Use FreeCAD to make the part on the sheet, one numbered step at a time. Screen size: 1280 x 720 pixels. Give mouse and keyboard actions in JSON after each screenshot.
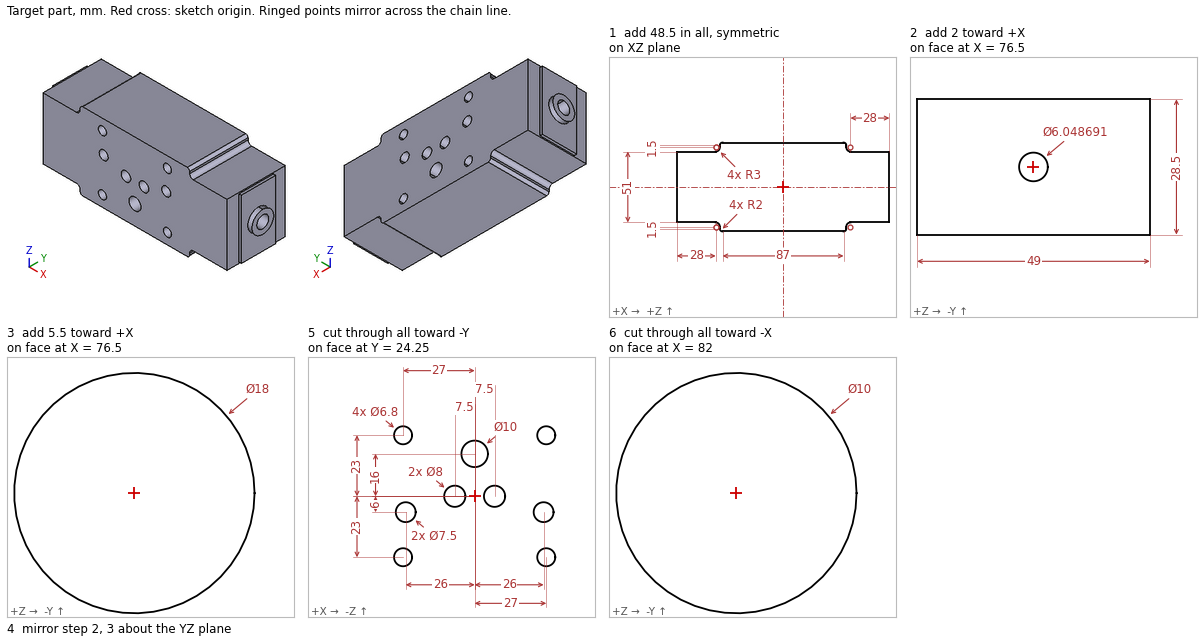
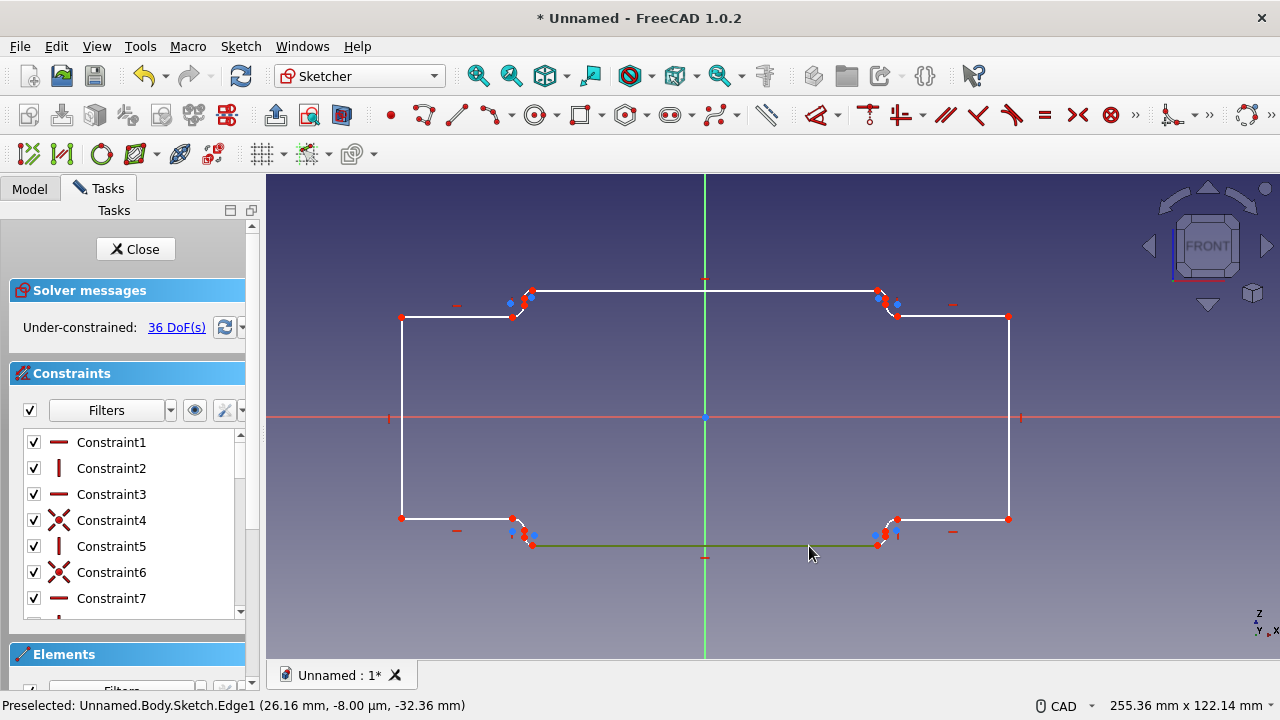
{"action": "scroll", "coordinate": [527, 543], "scroll_direction": "up", "scroll_amount": 4}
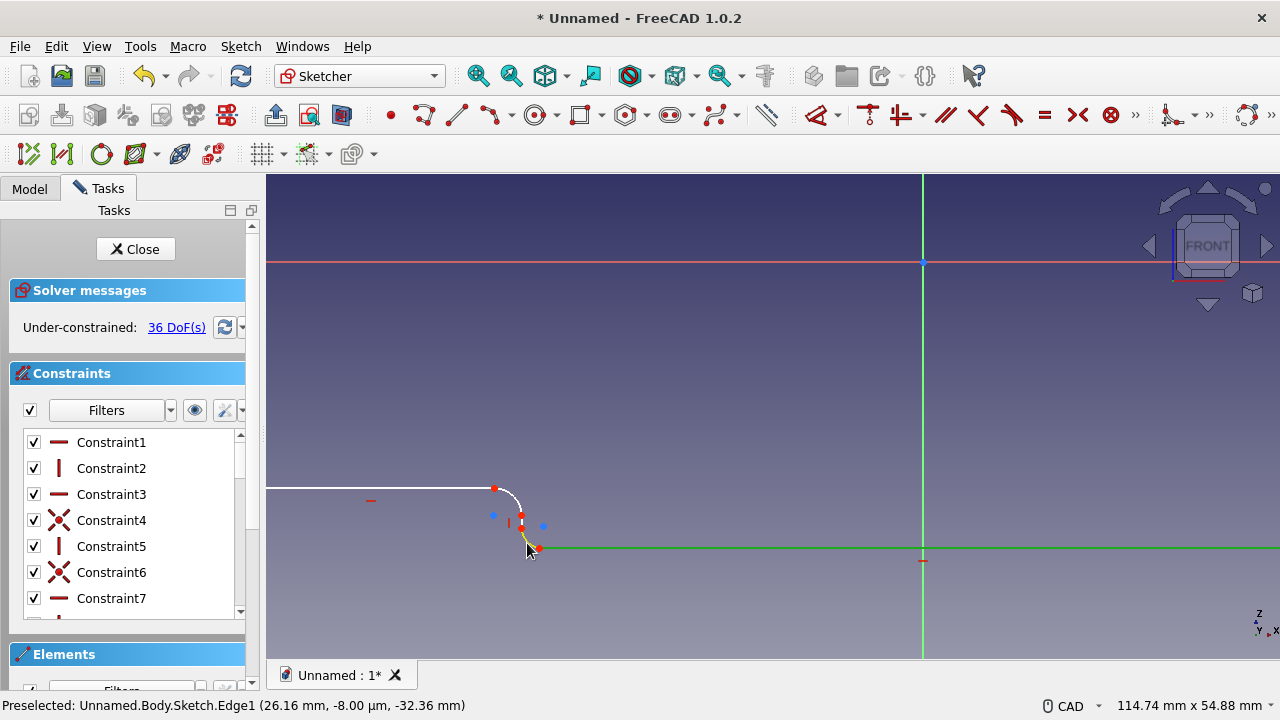
{"action": "left_click", "coordinate": [527, 541]}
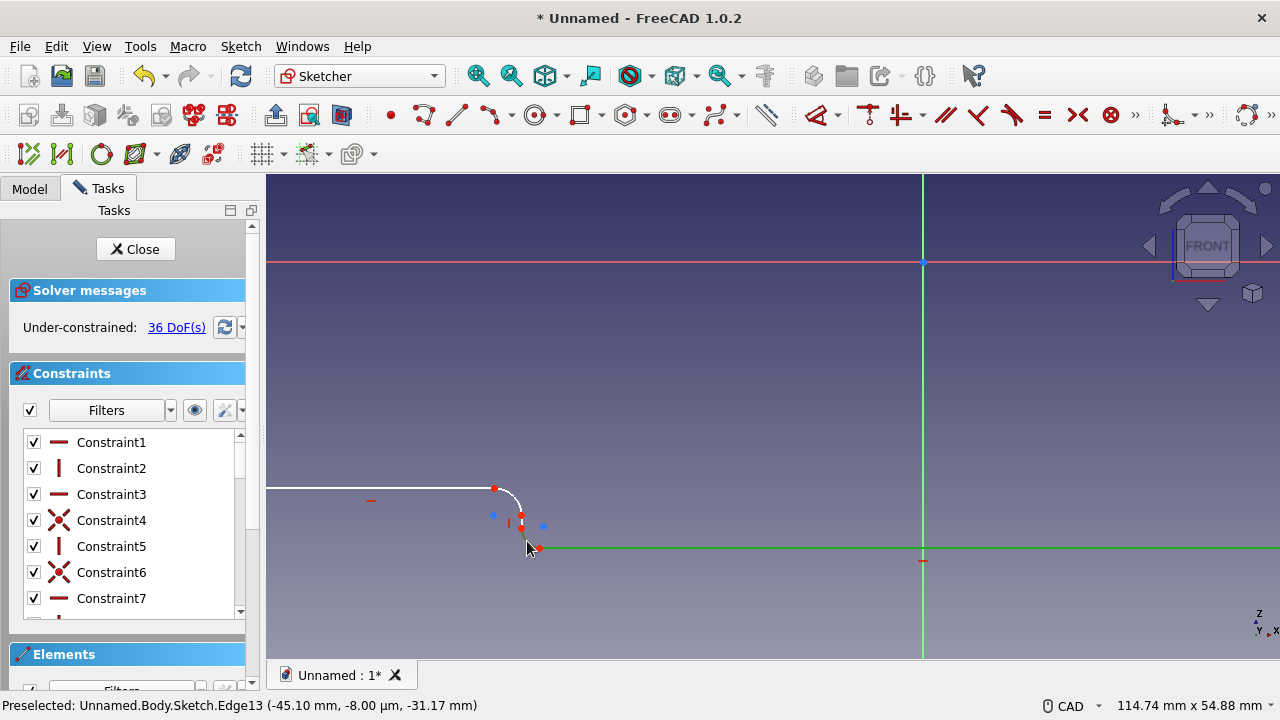
{"action": "left_click", "coordinate": [1012, 116]}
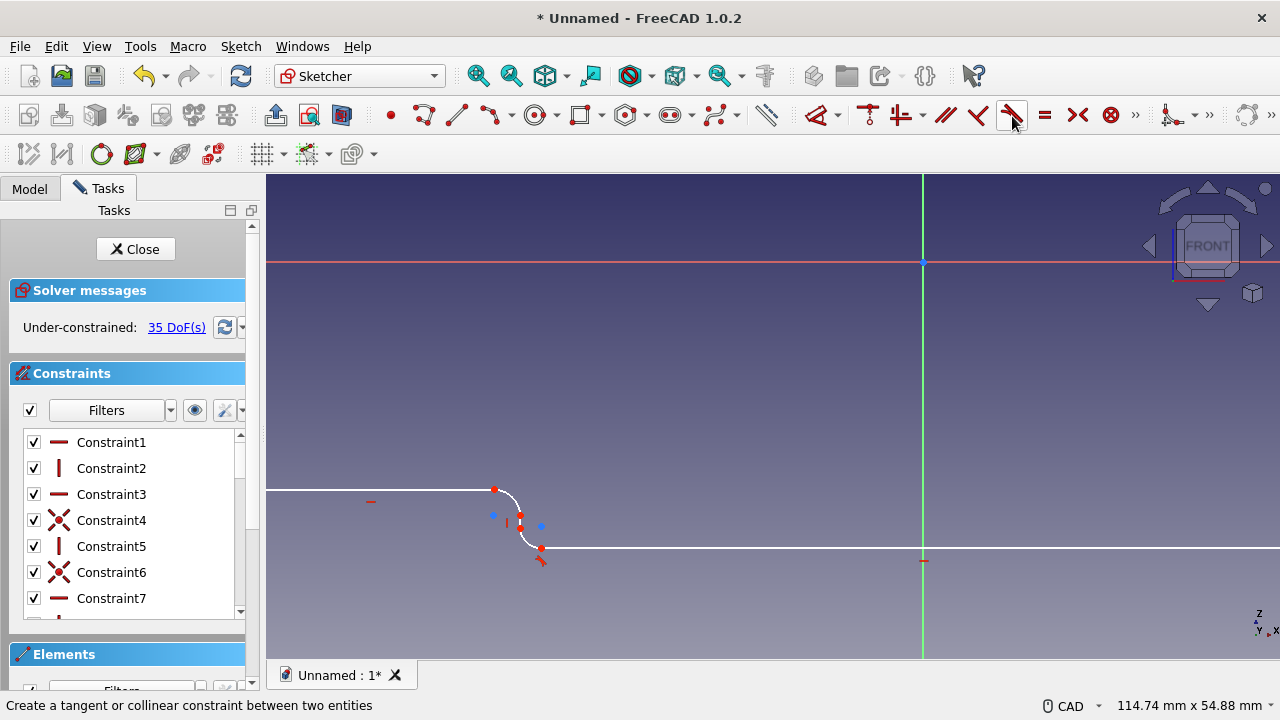
{"action": "left_click", "coordinate": [1077, 548]}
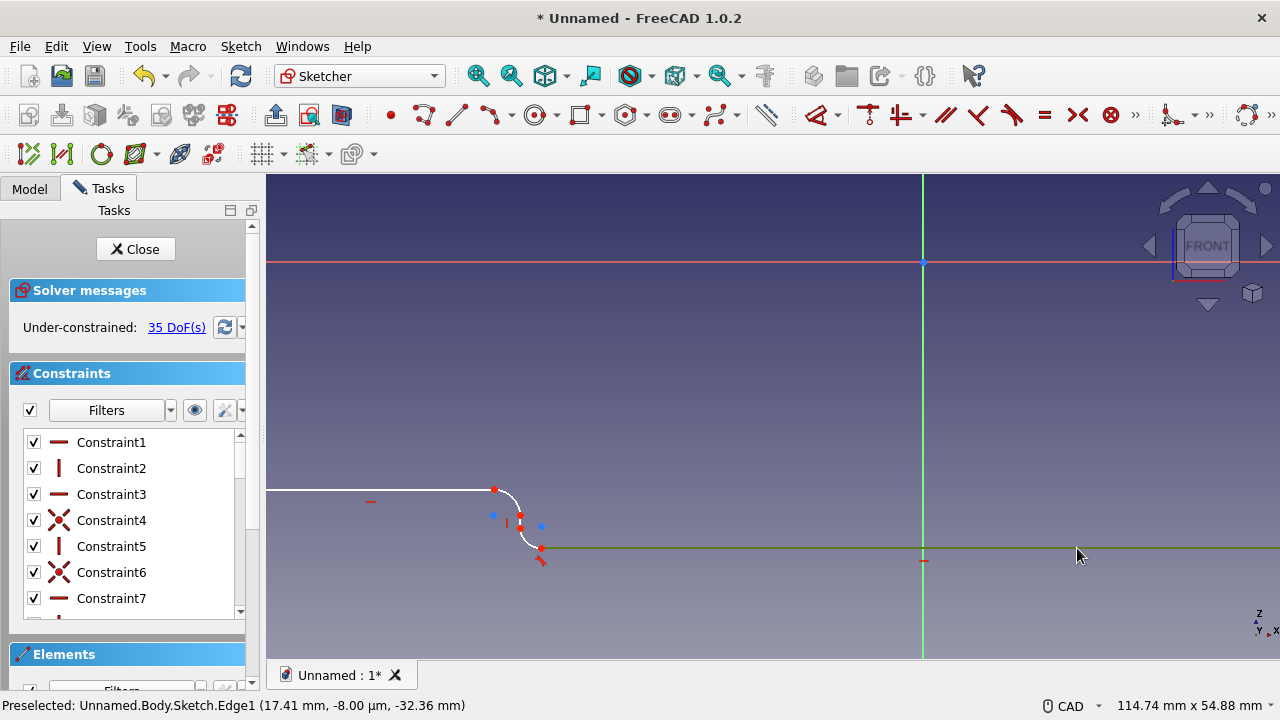
{"action": "scroll", "coordinate": [526, 542], "scroll_direction": "down", "scroll_amount": 4}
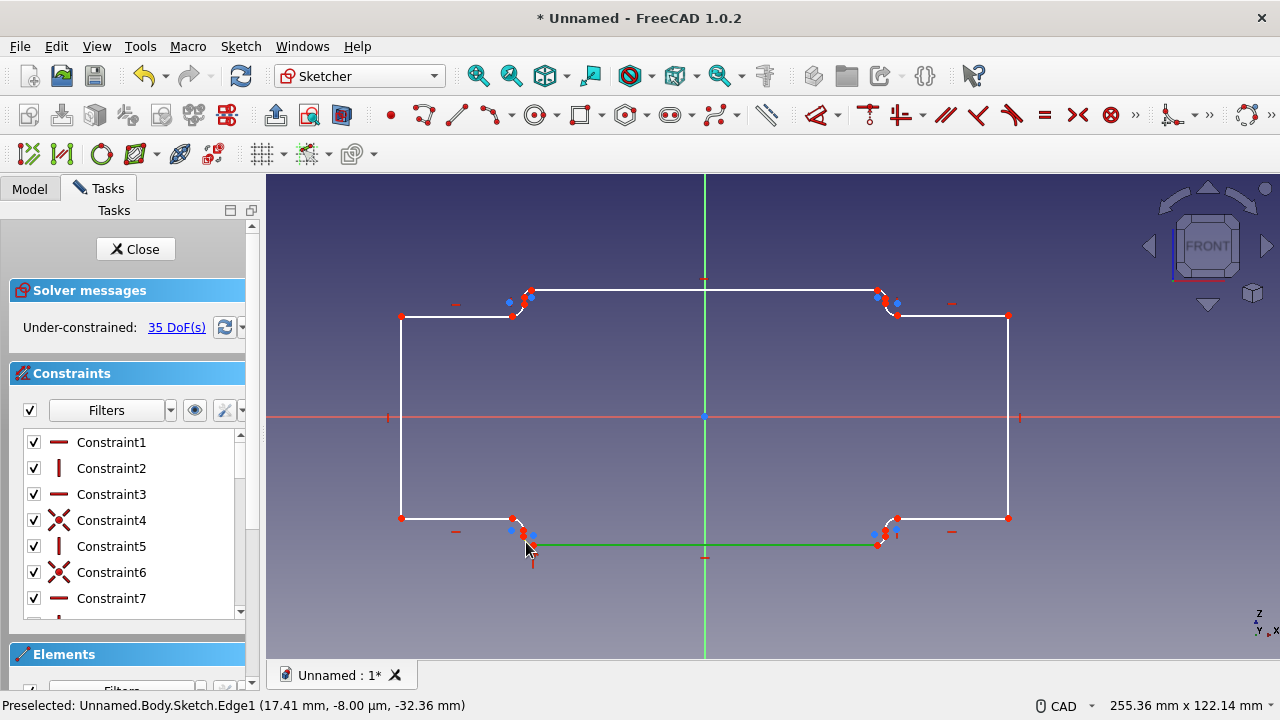
{"action": "scroll", "coordinate": [883, 542], "scroll_direction": "up", "scroll_amount": 4}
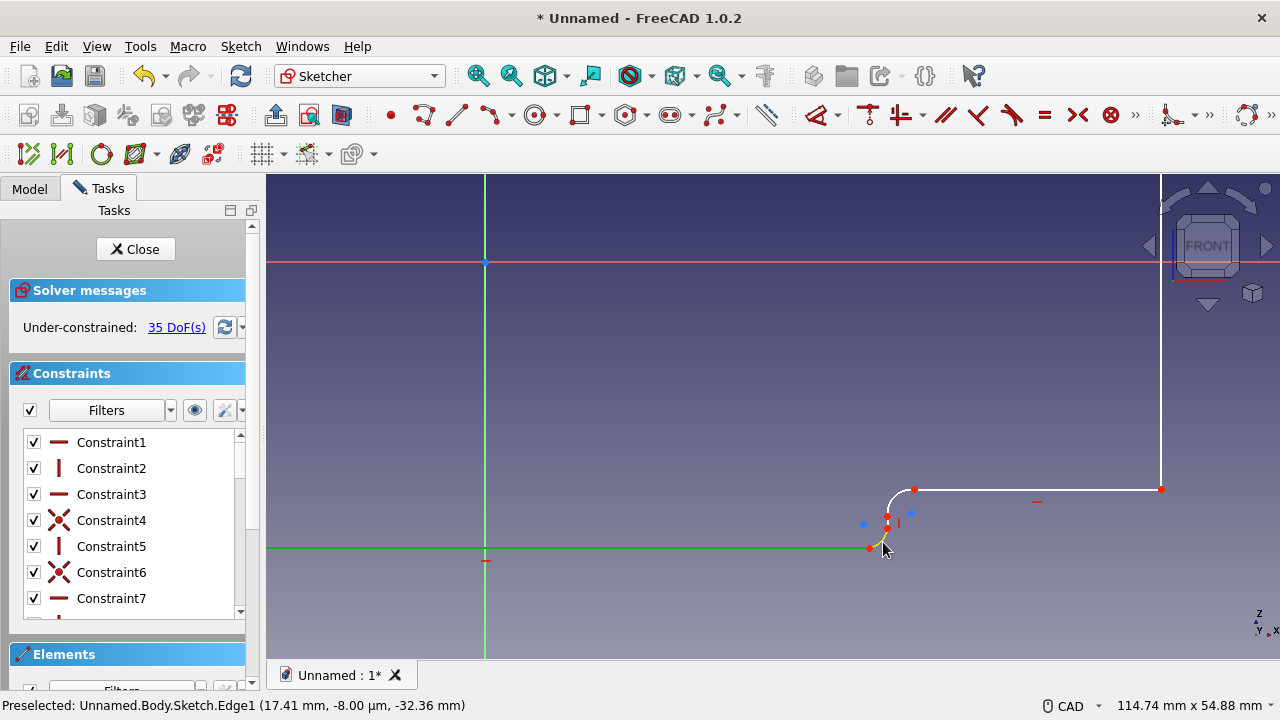
{"action": "left_click", "coordinate": [881, 541]}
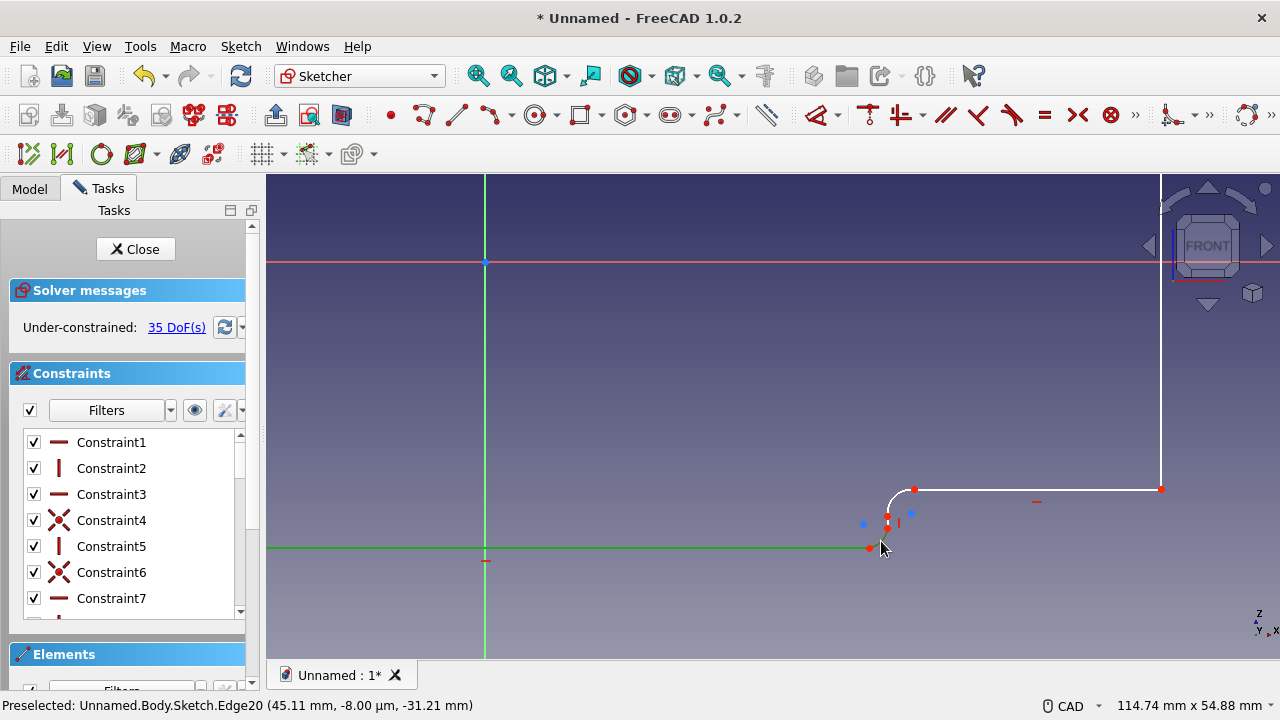
{"action": "key", "text": "t"}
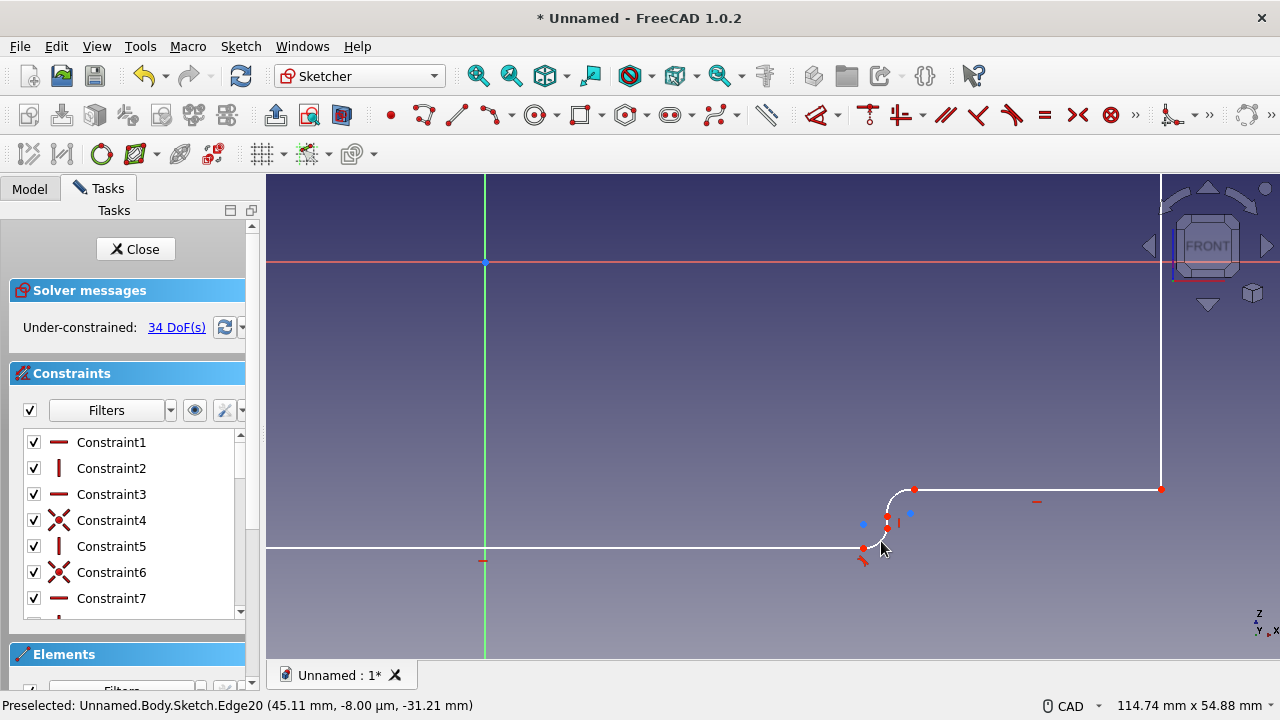
{"action": "scroll", "coordinate": [883, 542], "scroll_direction": "down", "scroll_amount": 4}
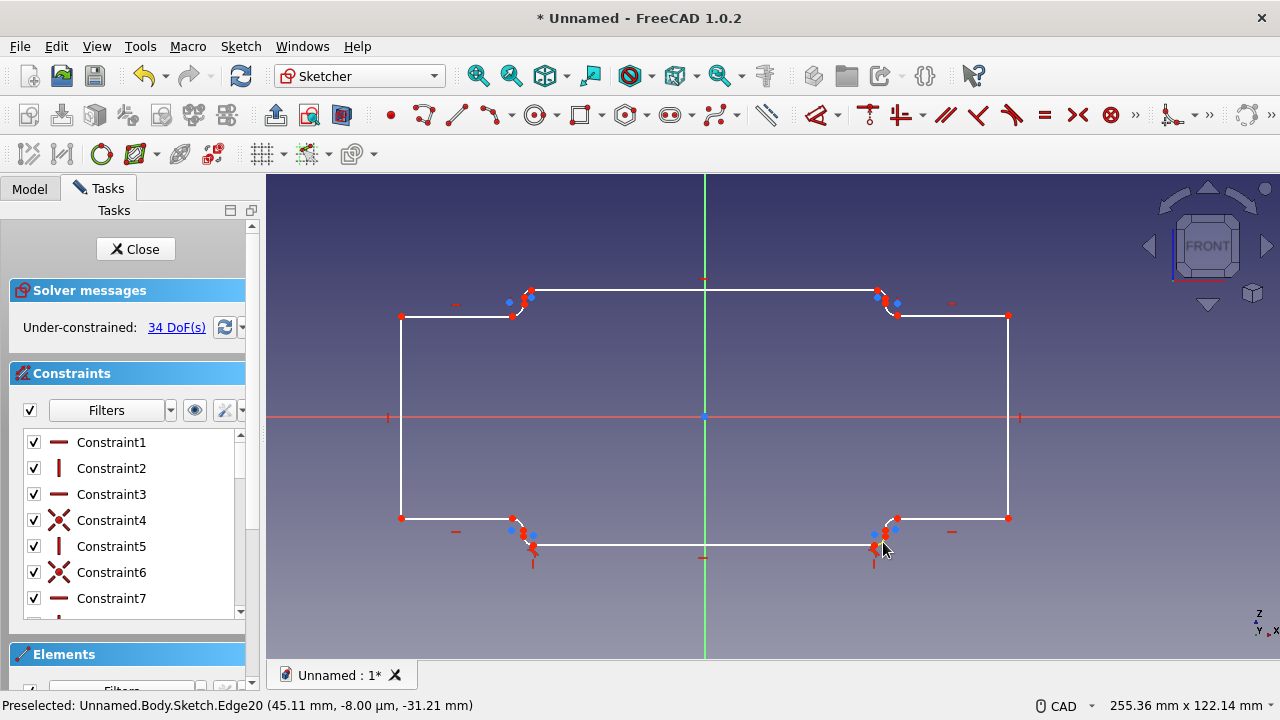
{"action": "scroll", "coordinate": [523, 533], "scroll_direction": "up", "scroll_amount": 8}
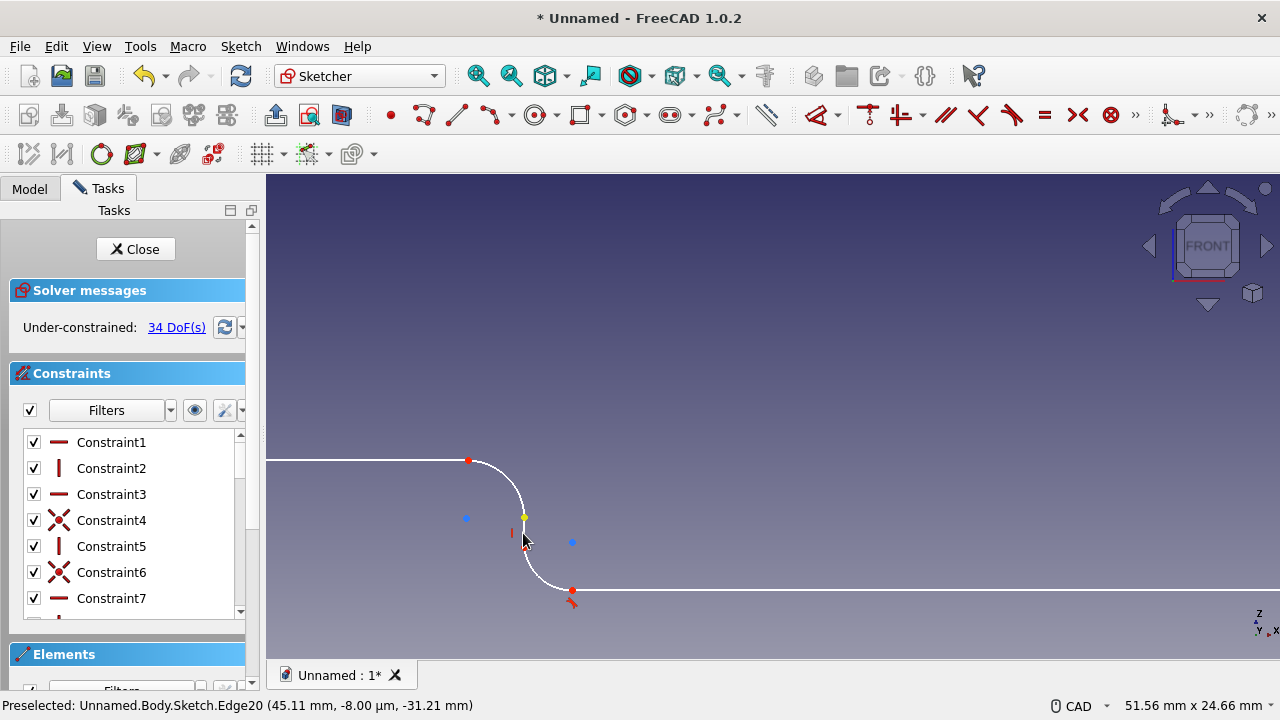
{"action": "left_click", "coordinate": [524, 532]}